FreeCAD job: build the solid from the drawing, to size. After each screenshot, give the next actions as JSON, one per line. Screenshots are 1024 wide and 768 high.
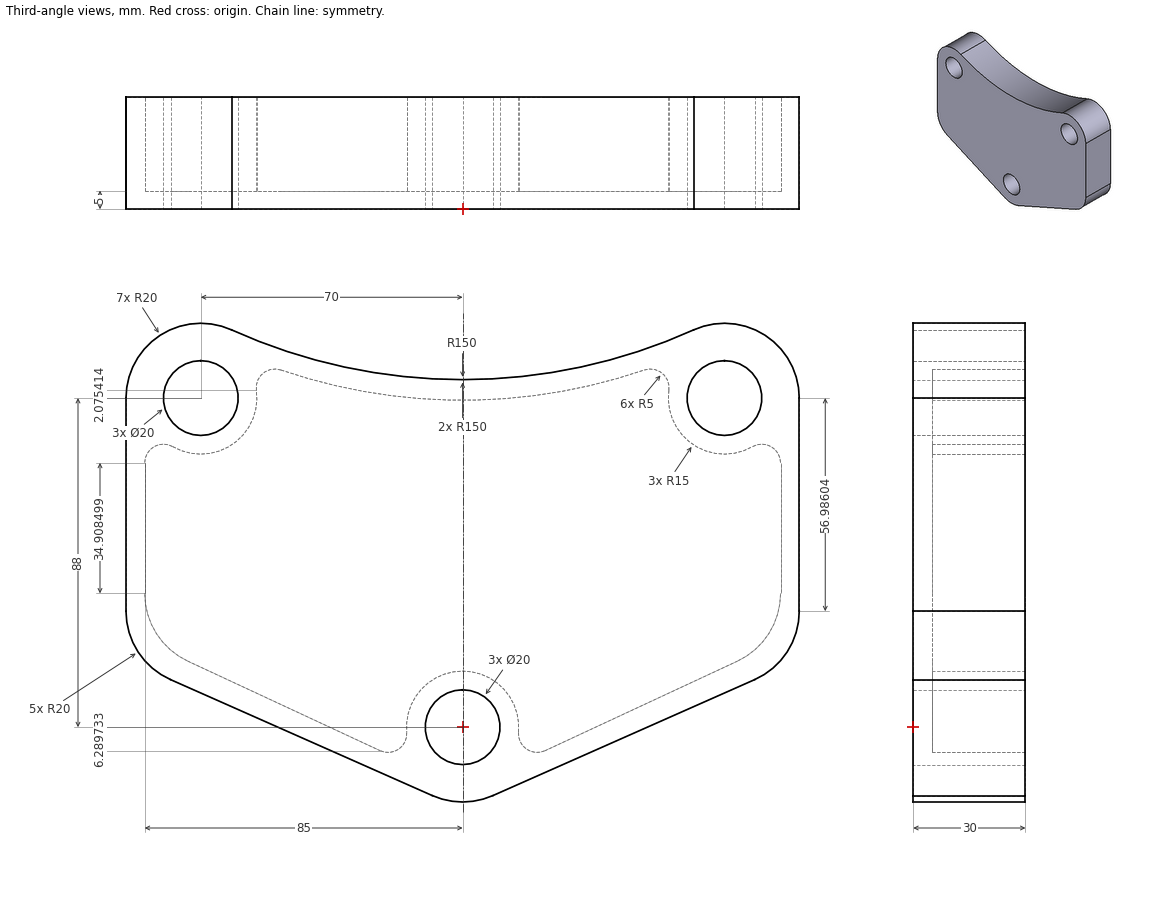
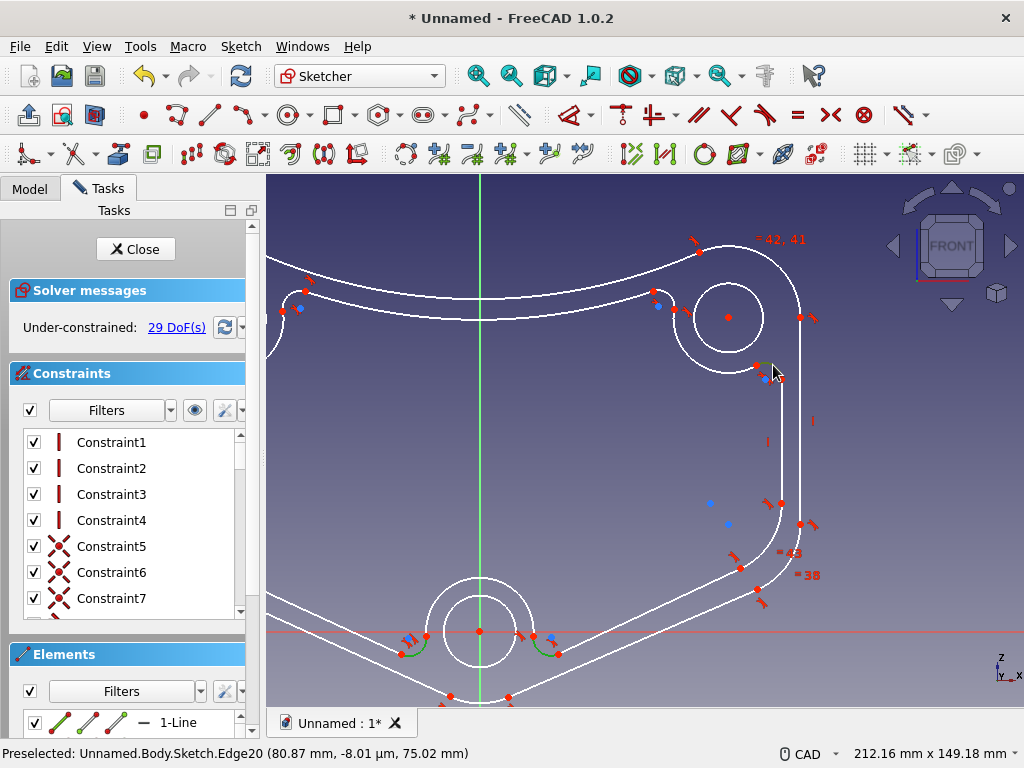
{"action": "scroll", "coordinate": [673, 299], "scroll_direction": "up", "scroll_amount": 2}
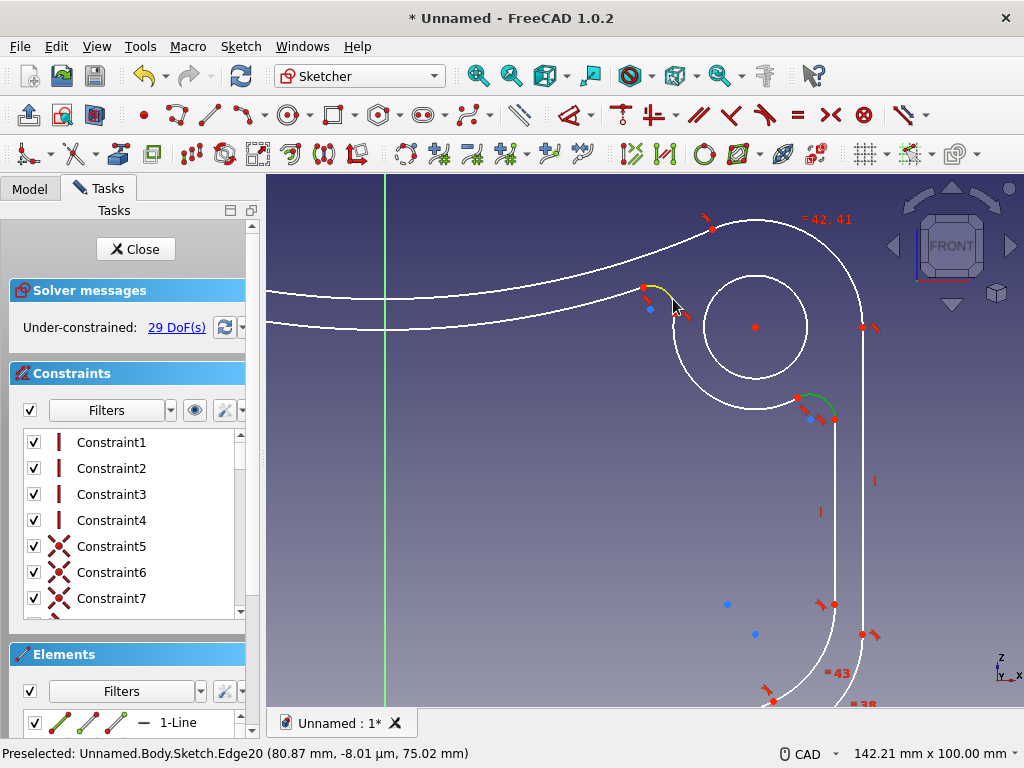
{"action": "left_click", "coordinate": [672, 299]}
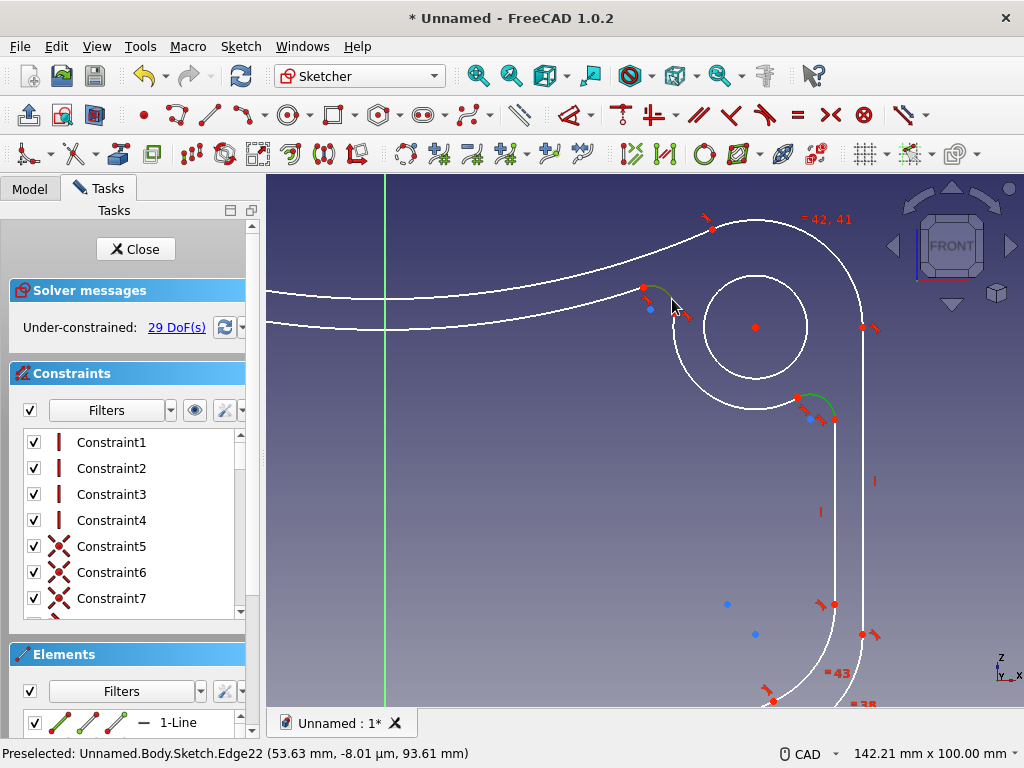
{"action": "scroll", "coordinate": [733, 339], "scroll_direction": "down", "scroll_amount": 4}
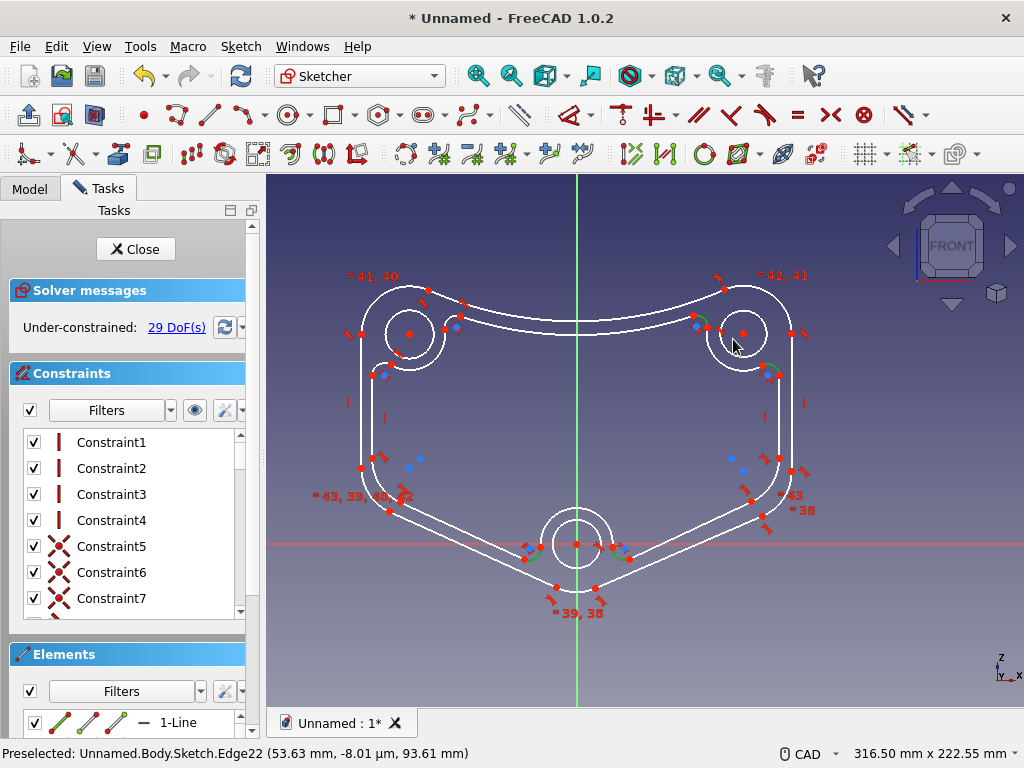
{"action": "scroll", "coordinate": [453, 316], "scroll_direction": "up", "scroll_amount": 4}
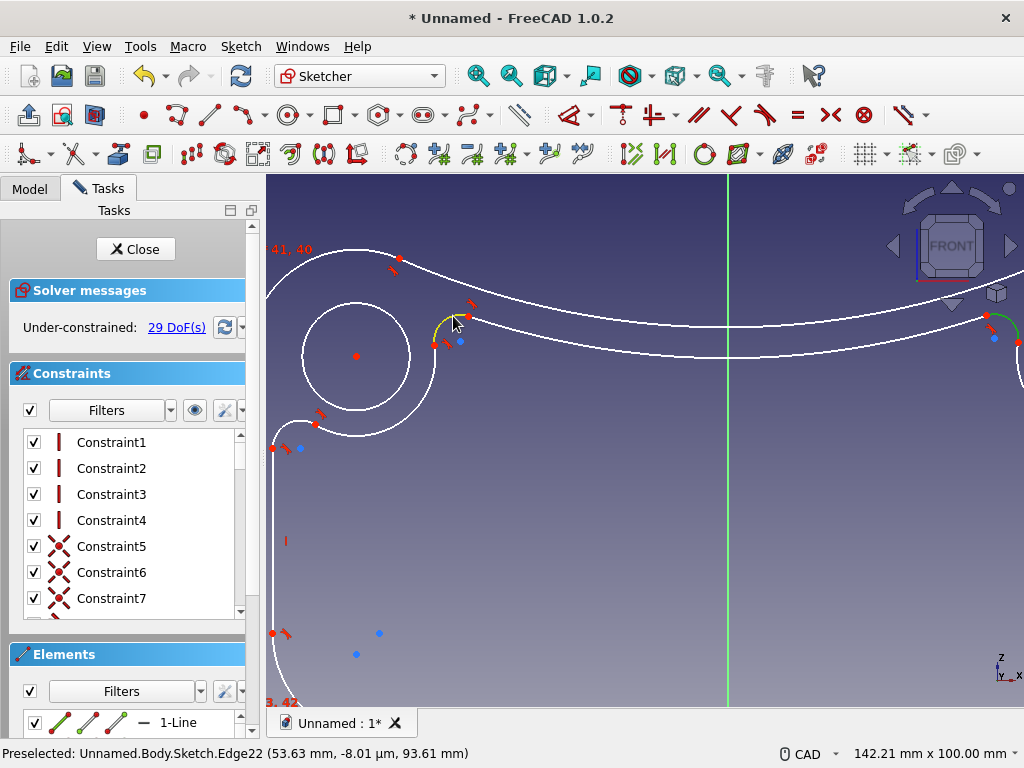
{"action": "left_click", "coordinate": [453, 316]}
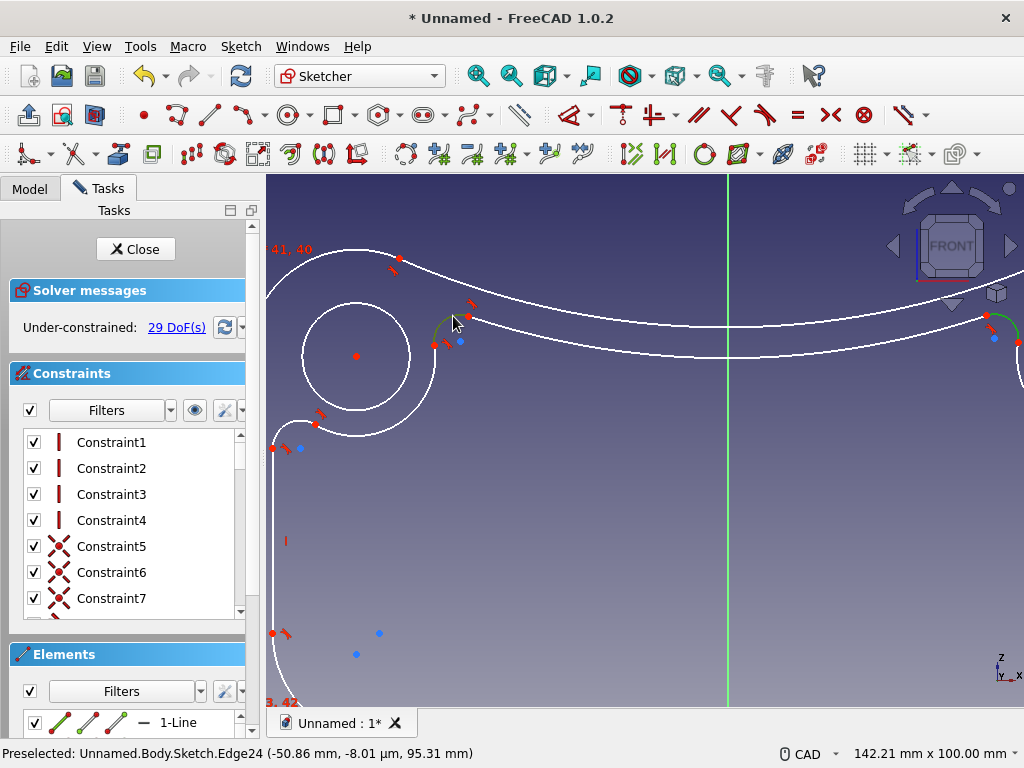
{"action": "left_click", "coordinate": [298, 421]}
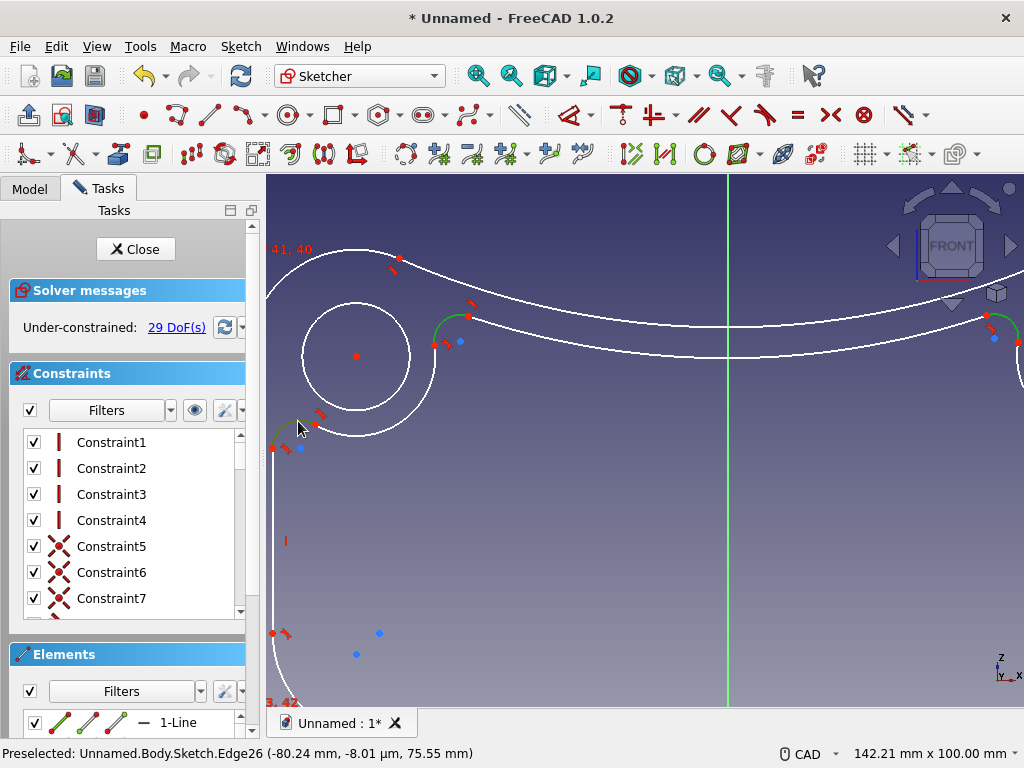
{"action": "left_click", "coordinate": [798, 116]}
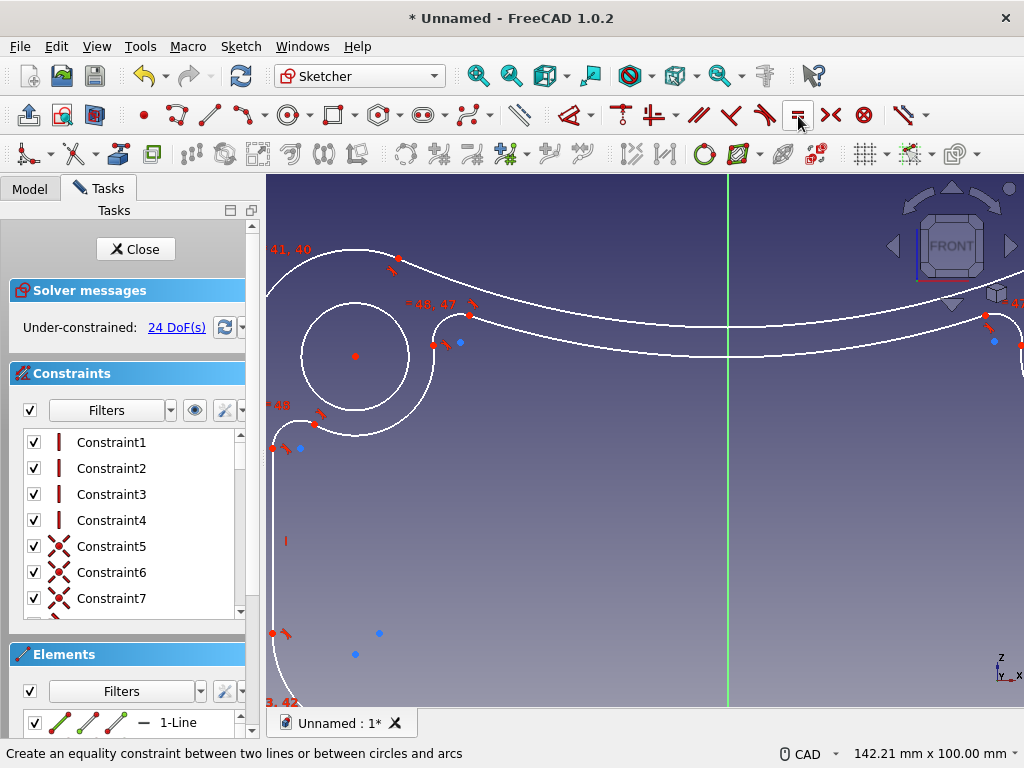
{"action": "scroll", "coordinate": [453, 316], "scroll_direction": "down", "scroll_amount": 4}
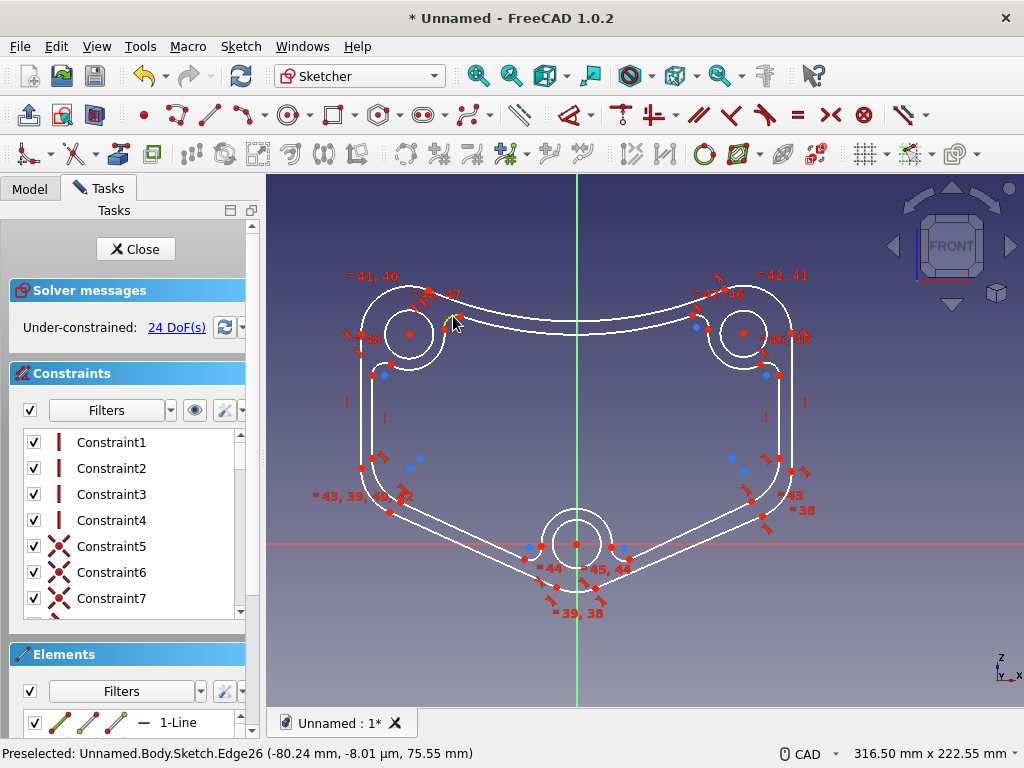
{"action": "scroll", "coordinate": [599, 516], "scroll_direction": "up", "scroll_amount": 2}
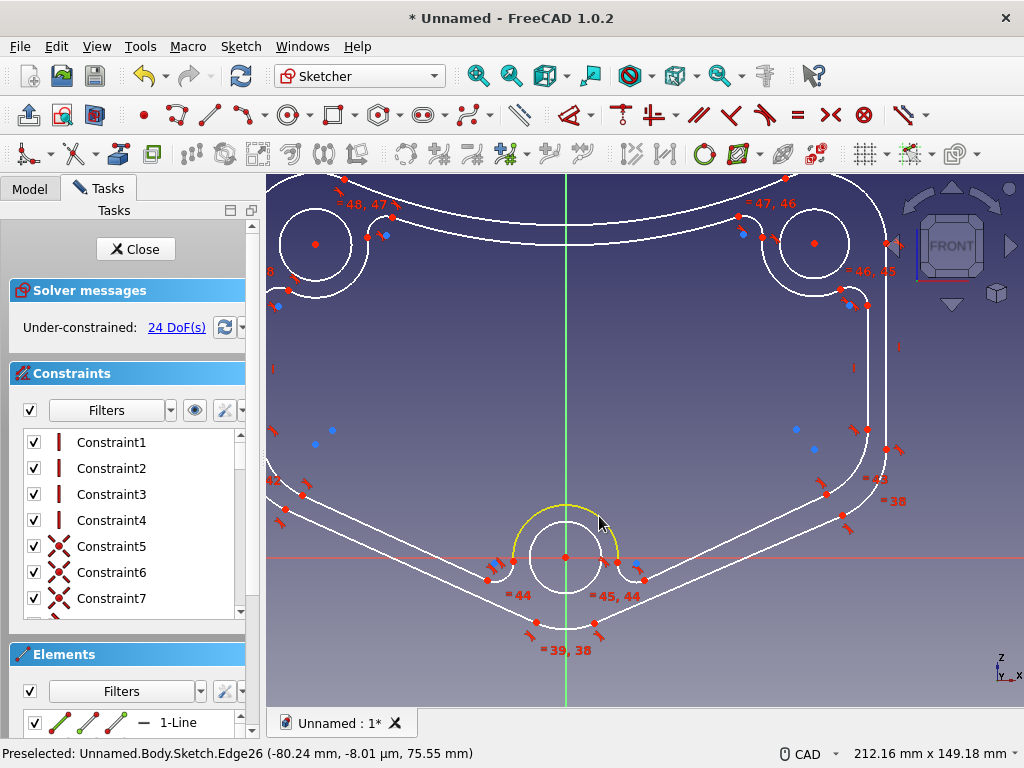
{"action": "left_click", "coordinate": [598, 516]}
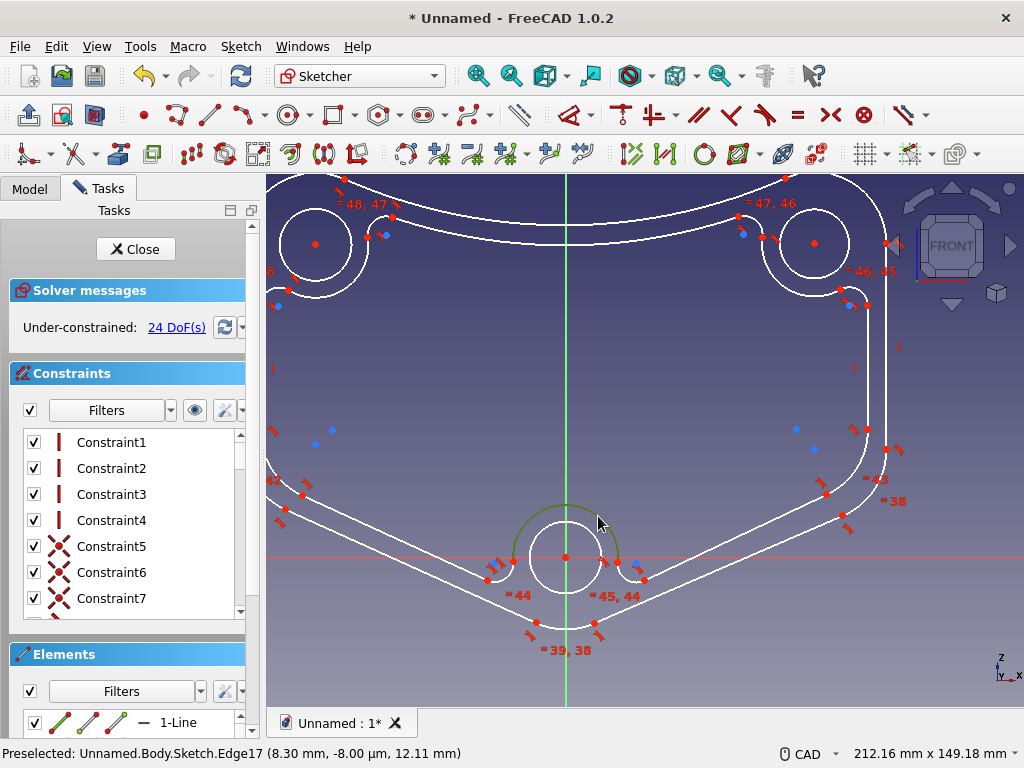
{"action": "left_click", "coordinate": [769, 271]}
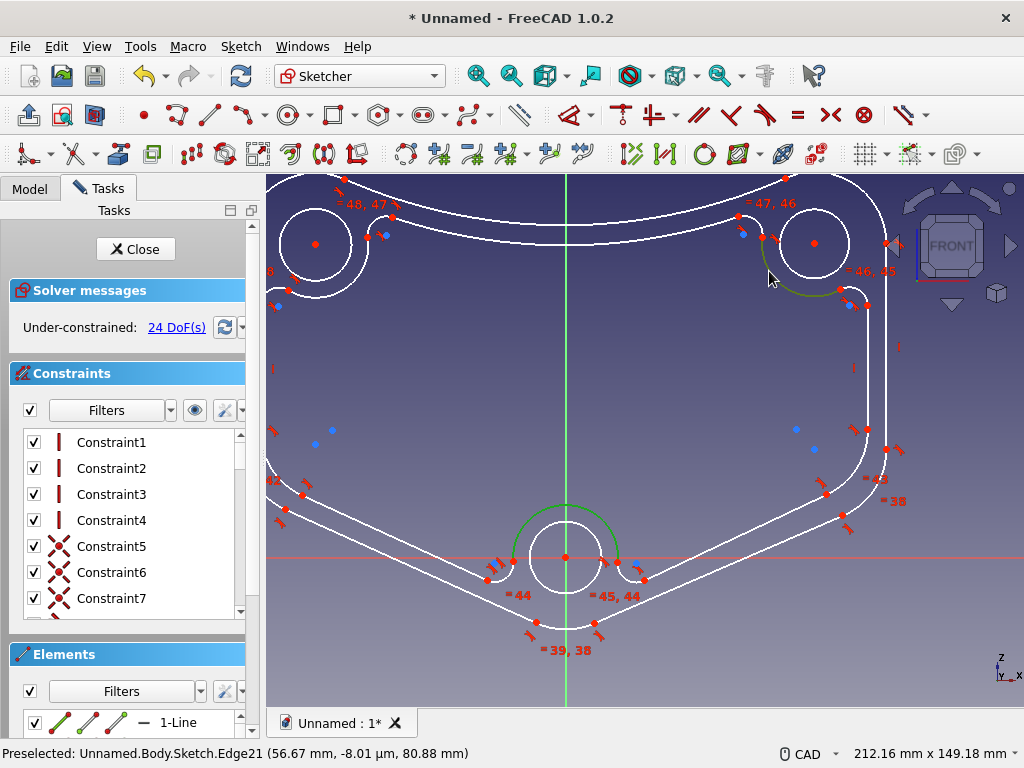
{"action": "left_click", "coordinate": [323, 297]}